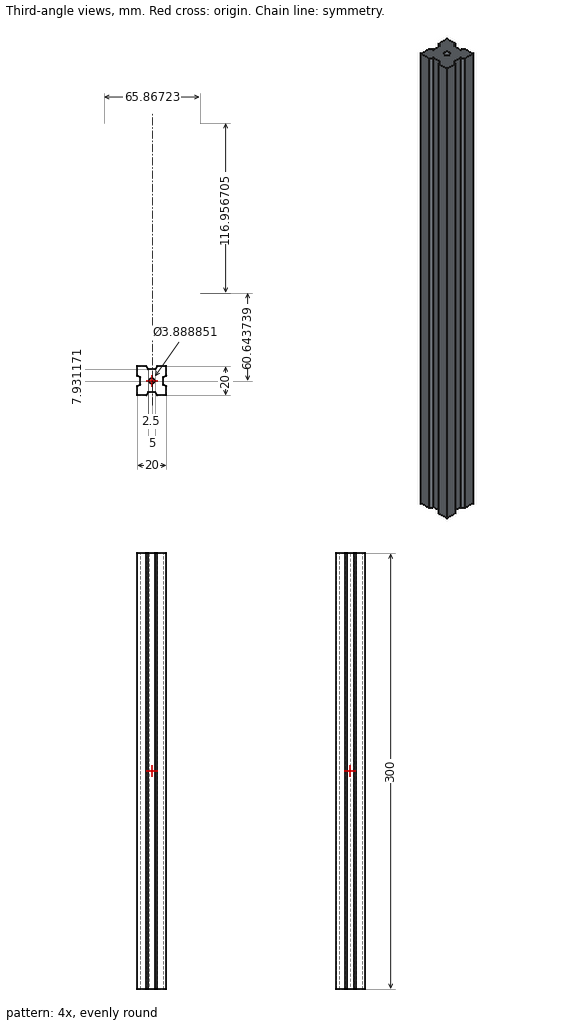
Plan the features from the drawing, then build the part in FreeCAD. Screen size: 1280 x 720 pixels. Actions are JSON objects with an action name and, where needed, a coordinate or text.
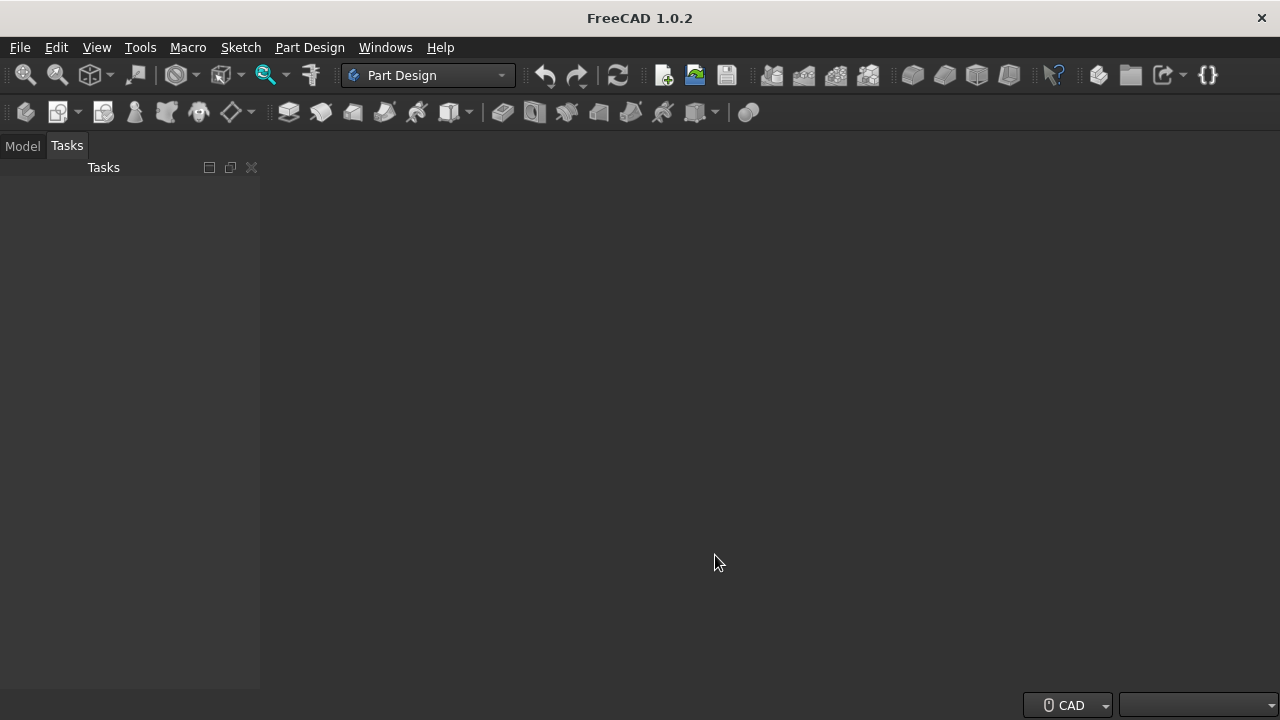
{"action": "key", "text": "ctrl+n"}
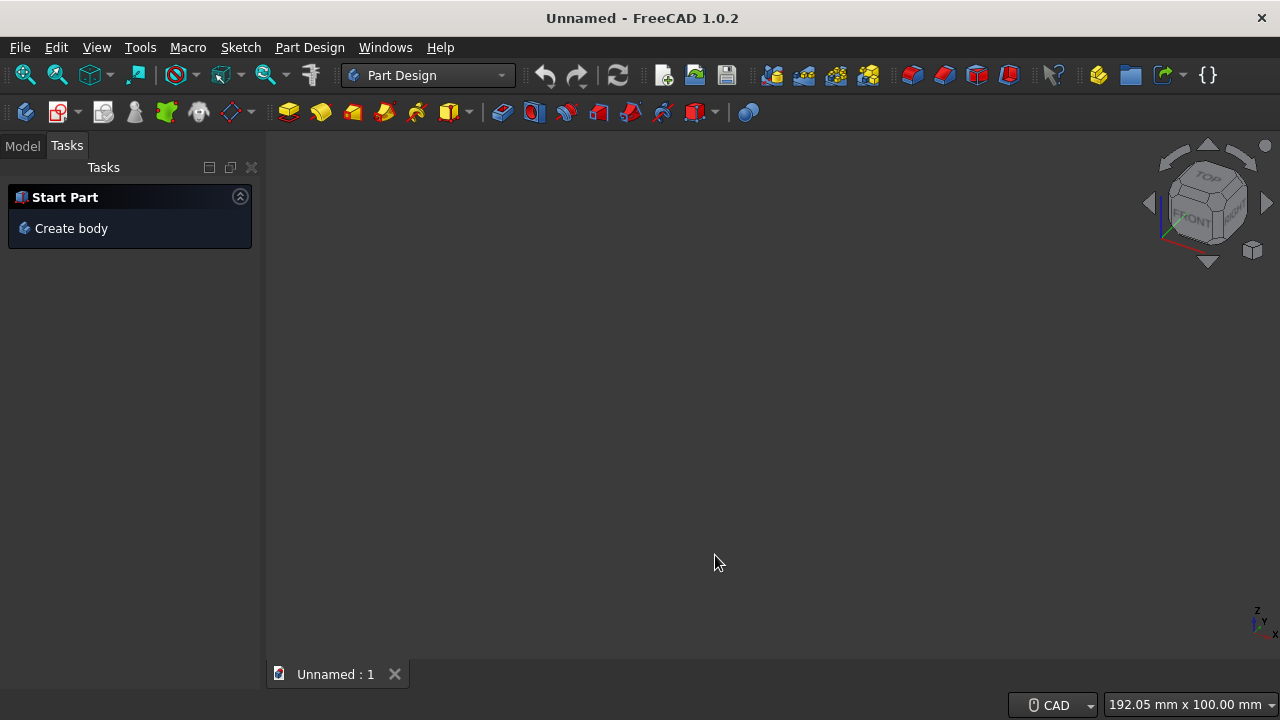
{"action": "left_click", "coordinate": [58, 112]}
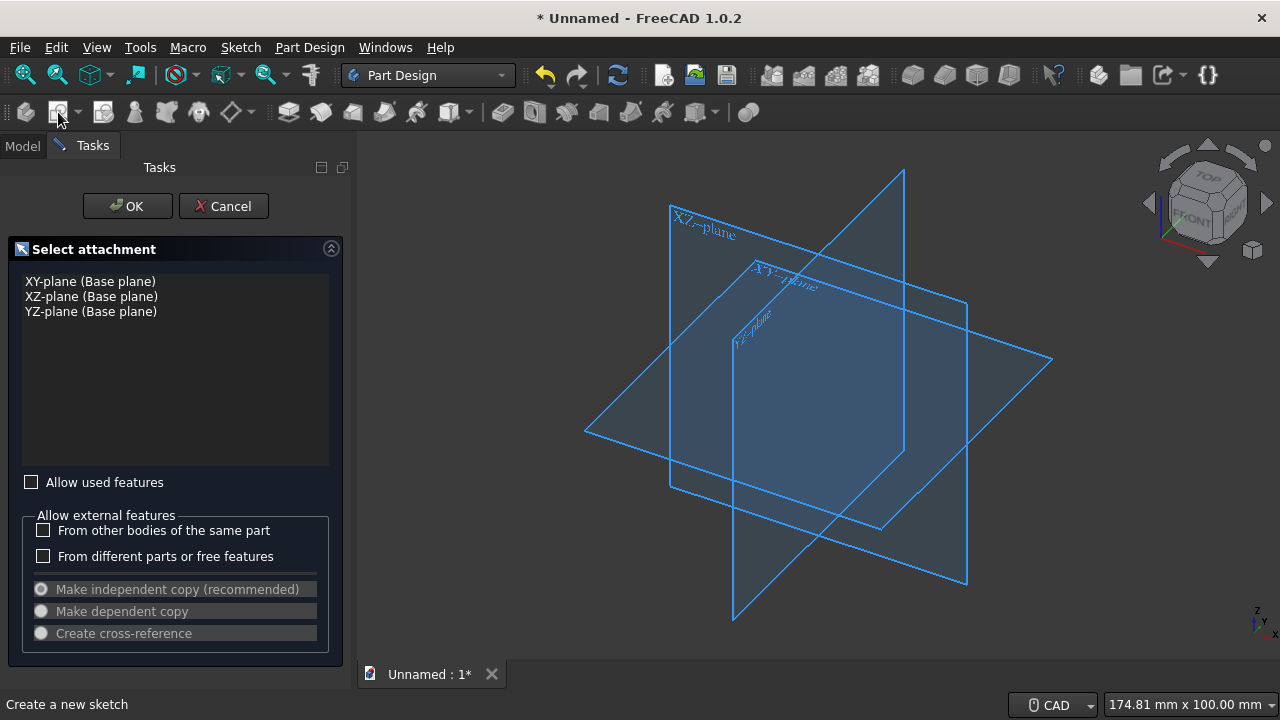
{"action": "left_click", "coordinate": [82, 282]}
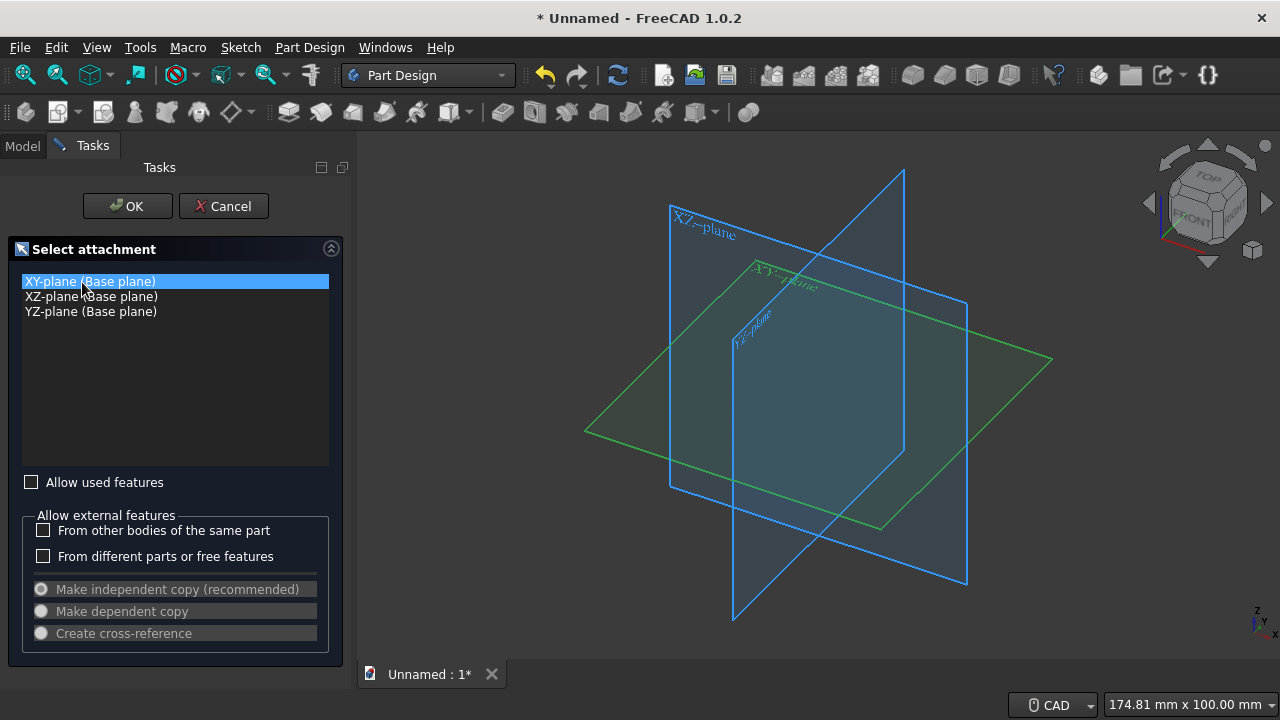
{"action": "left_click", "coordinate": [128, 206]}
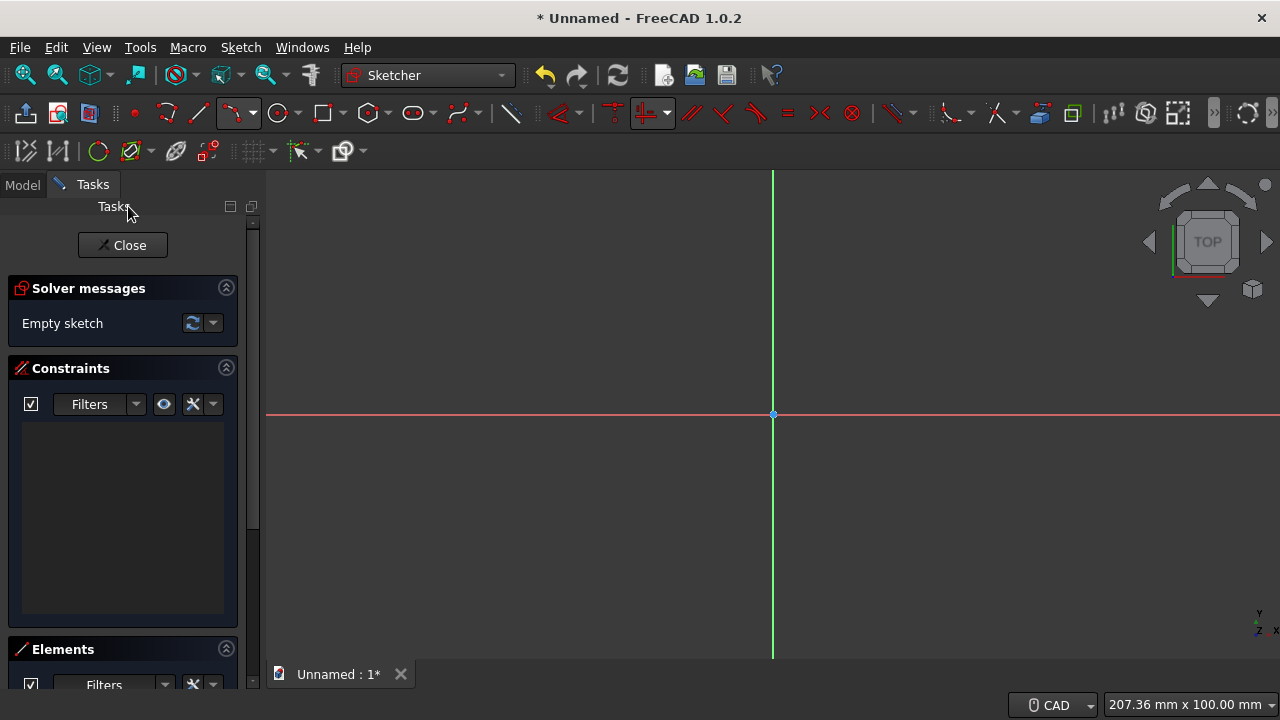
{"action": "scroll", "coordinate": [803, 415], "scroll_direction": "up", "scroll_amount": 6}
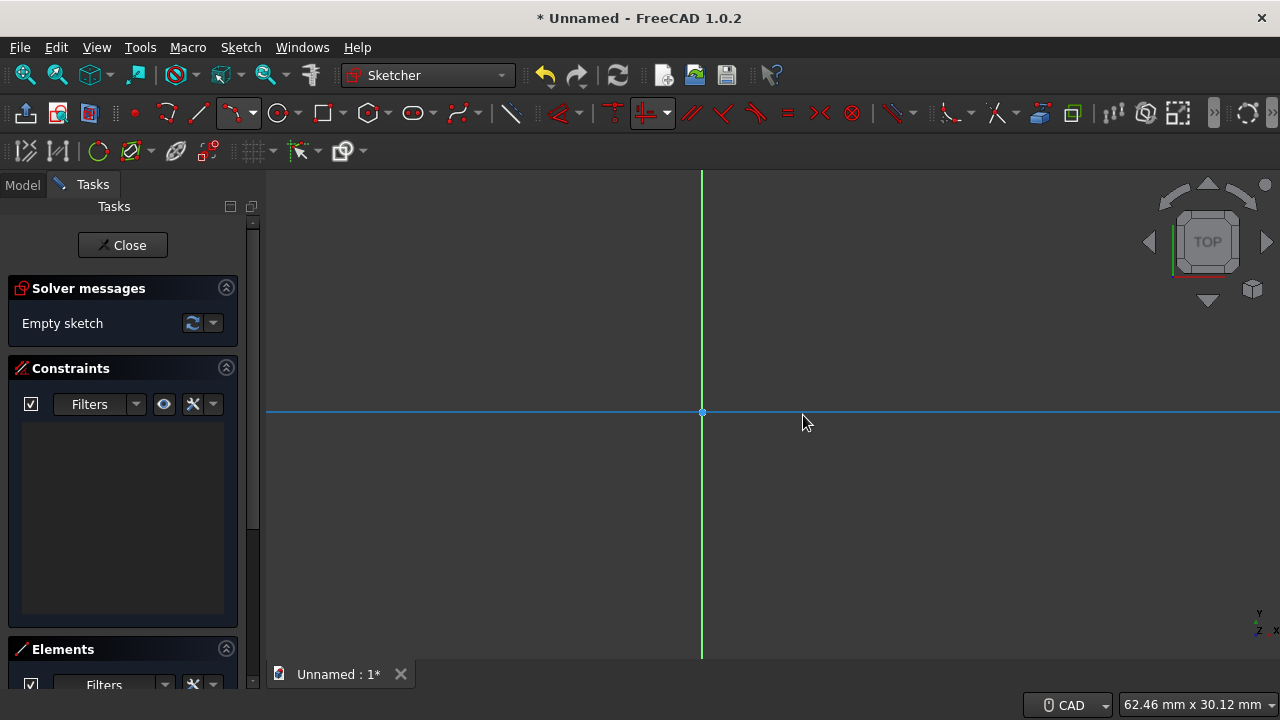
{"action": "left_click", "coordinate": [346, 114]}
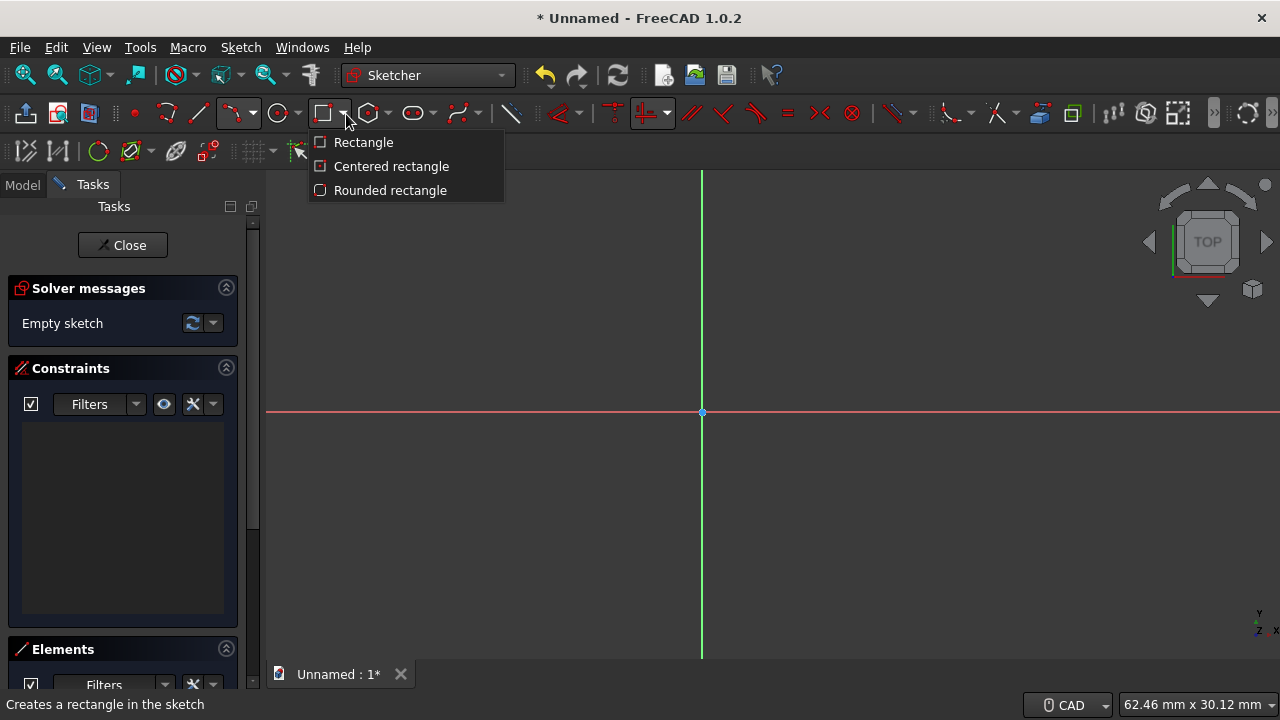
{"action": "left_click", "coordinate": [406, 166]}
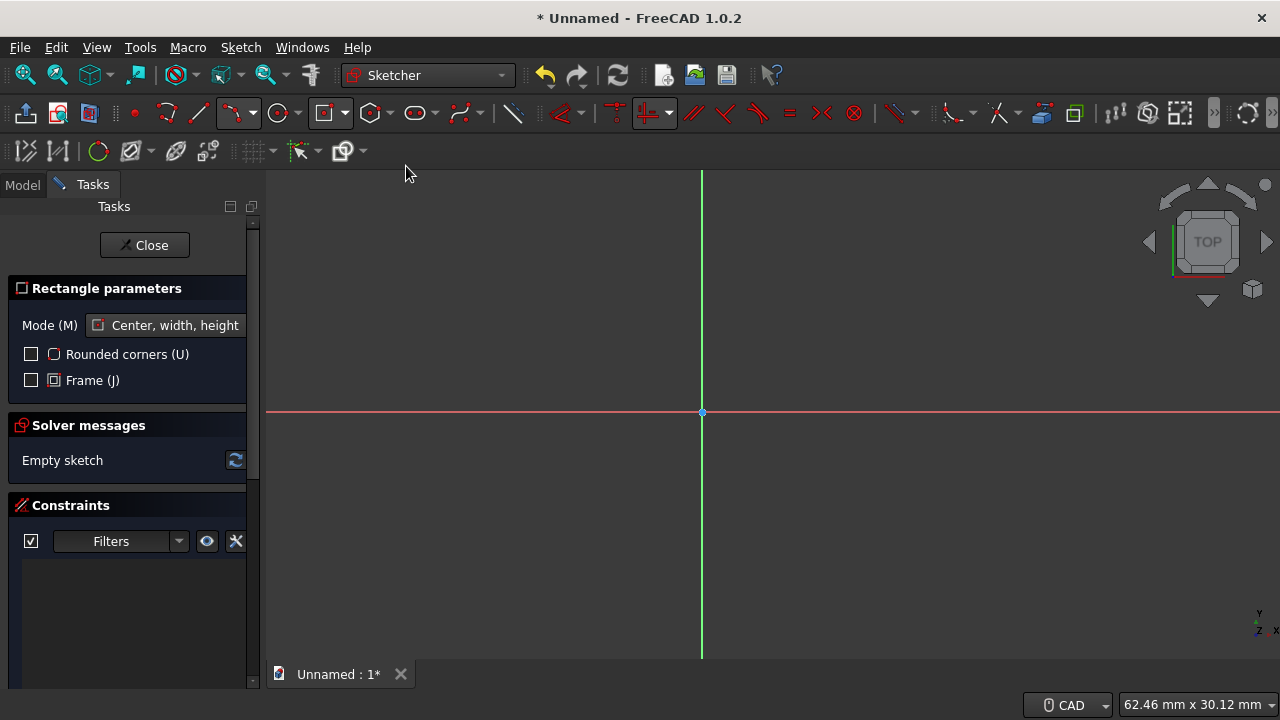
{"action": "left_click", "coordinate": [702, 412]}
{"action": "left_click", "coordinate": [865, 250]}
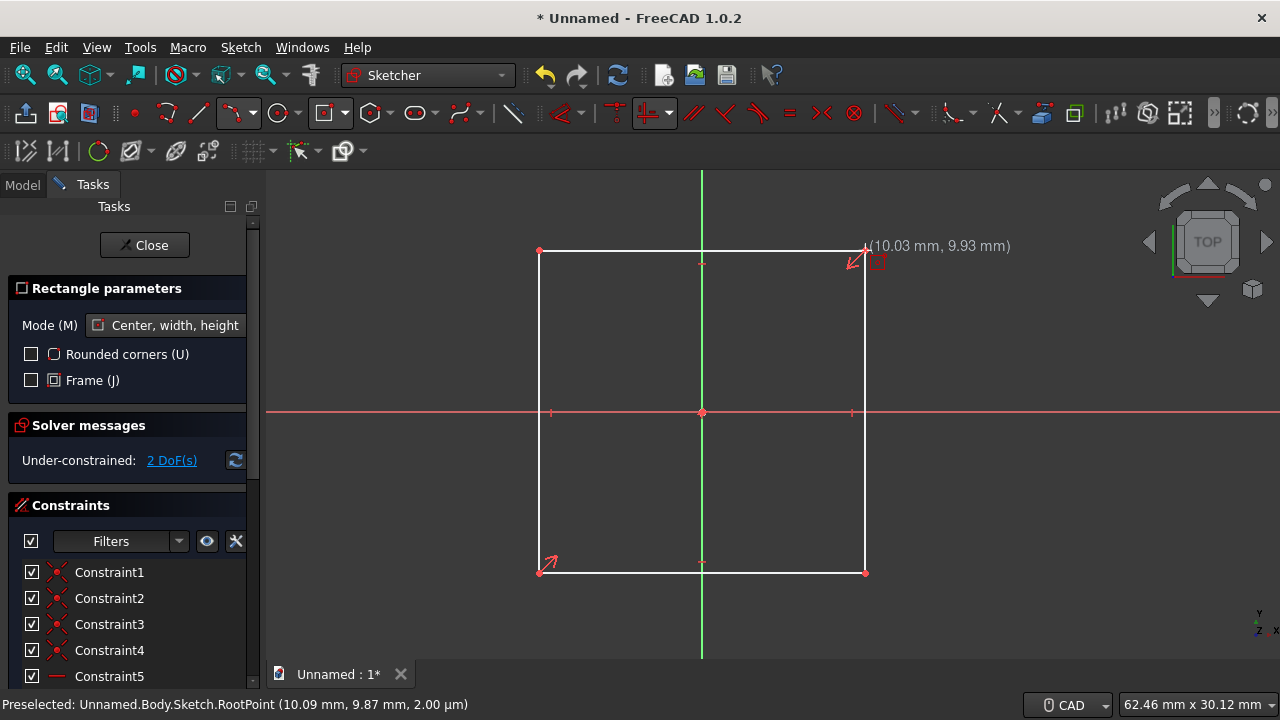
{"action": "left_click", "coordinate": [278, 114]}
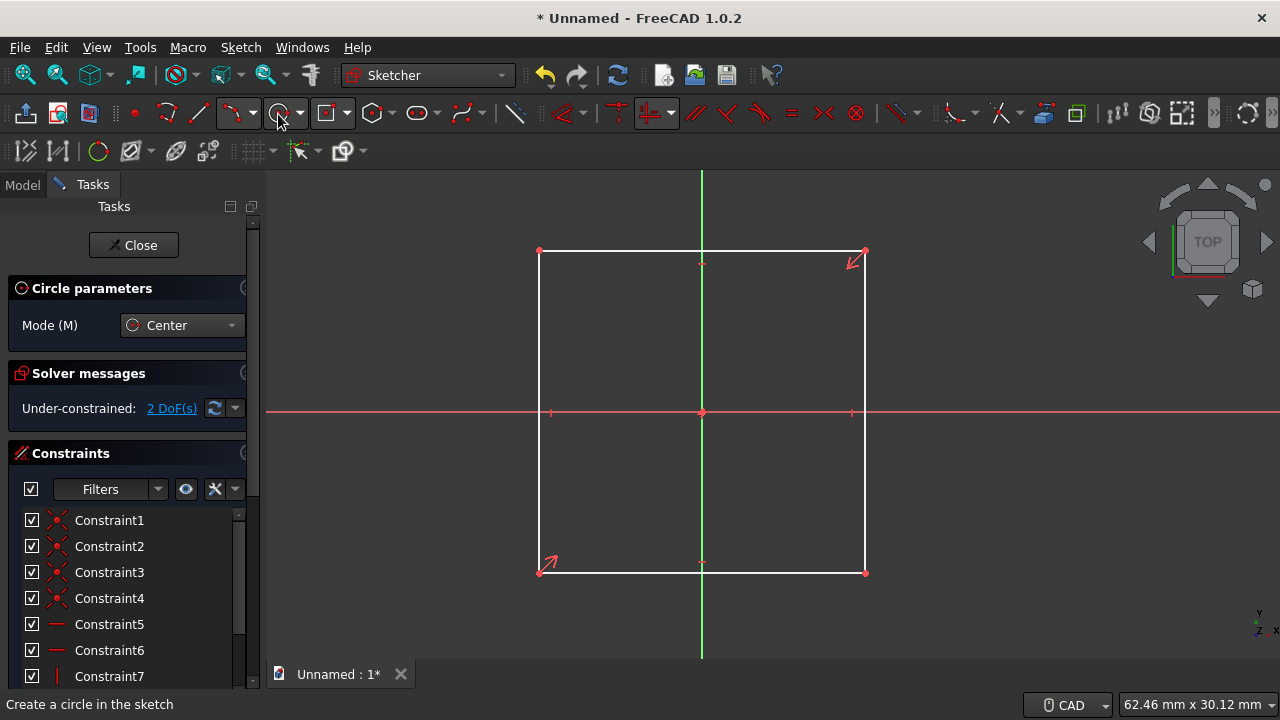
{"action": "left_click", "coordinate": [702, 412]}
{"action": "left_click", "coordinate": [724, 390]}
{"action": "key", "text": "Escape"}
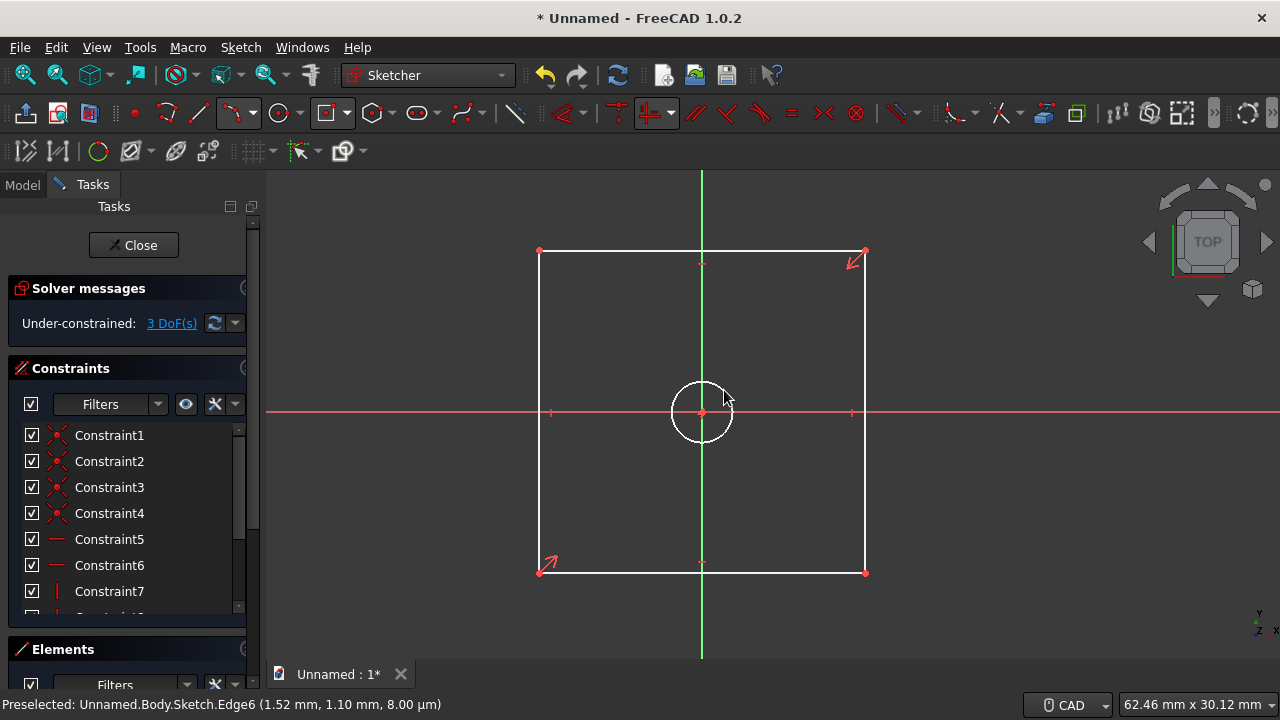
{"action": "left_click", "coordinate": [562, 114]}